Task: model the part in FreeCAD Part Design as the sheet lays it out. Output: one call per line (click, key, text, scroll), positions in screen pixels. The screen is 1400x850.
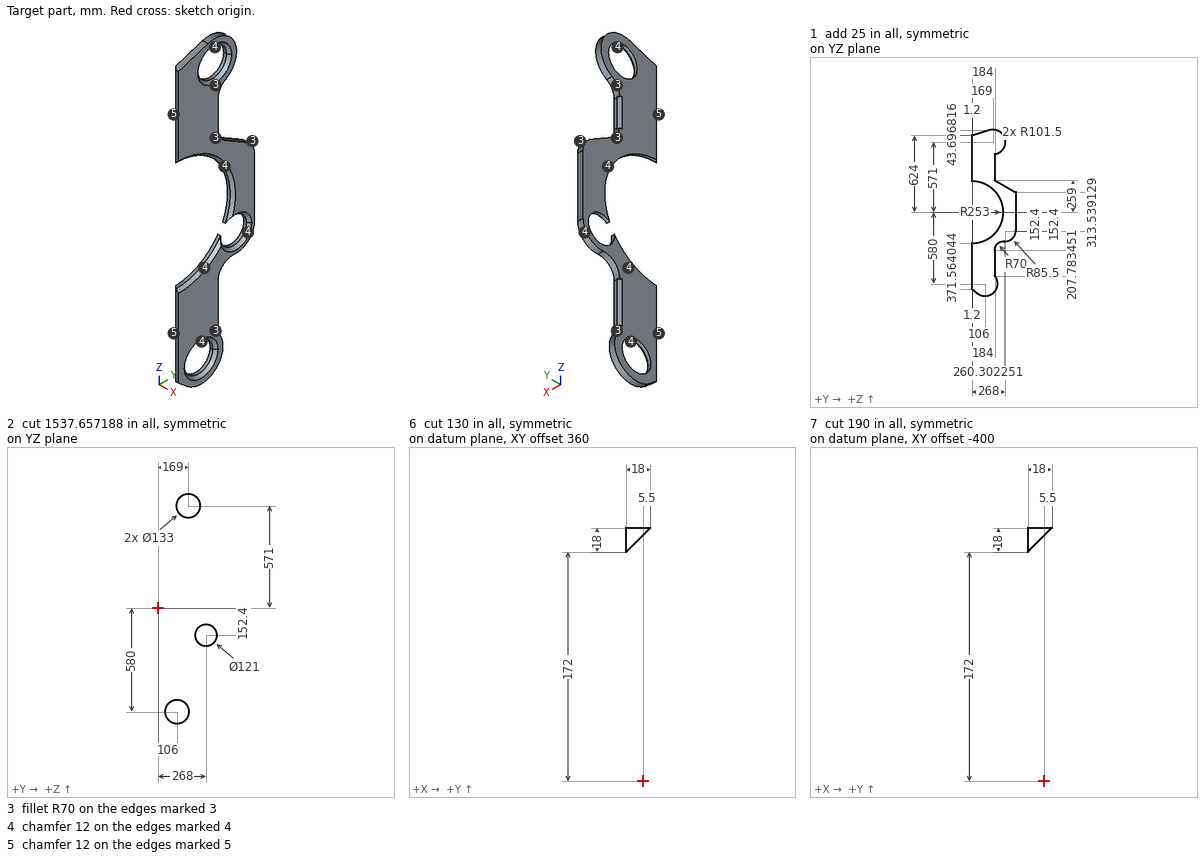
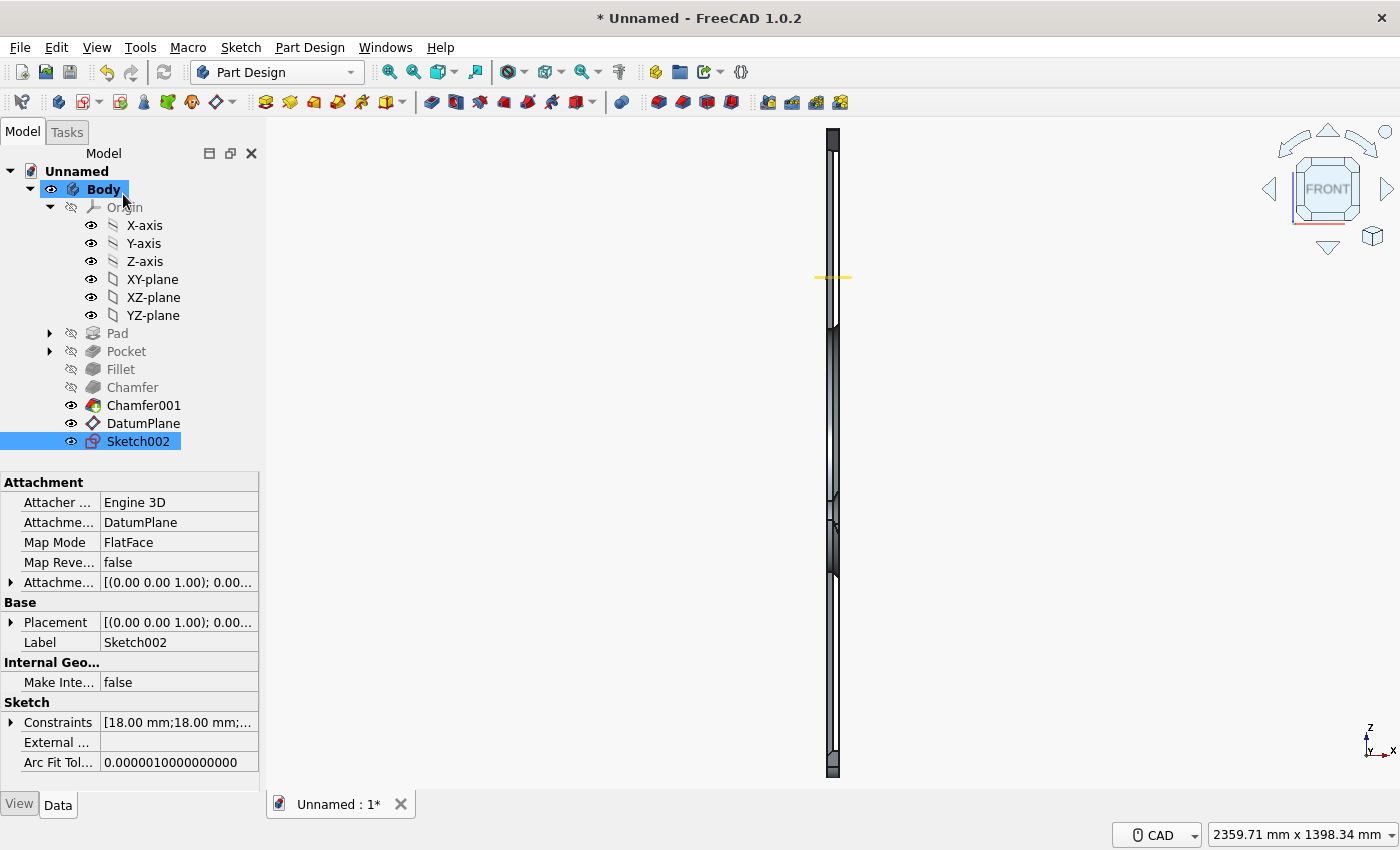
click(432, 102)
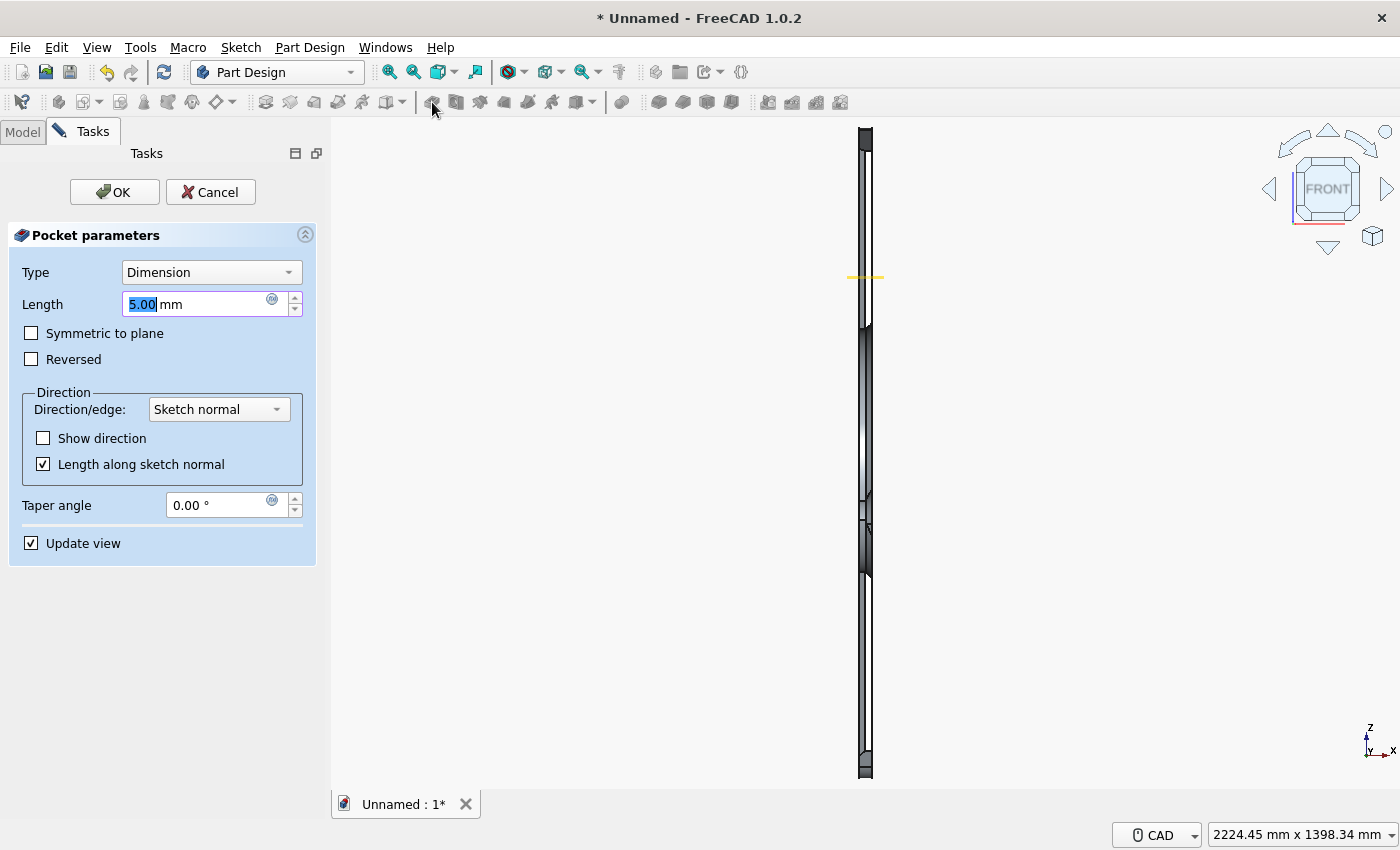
text(130)
key(Tab)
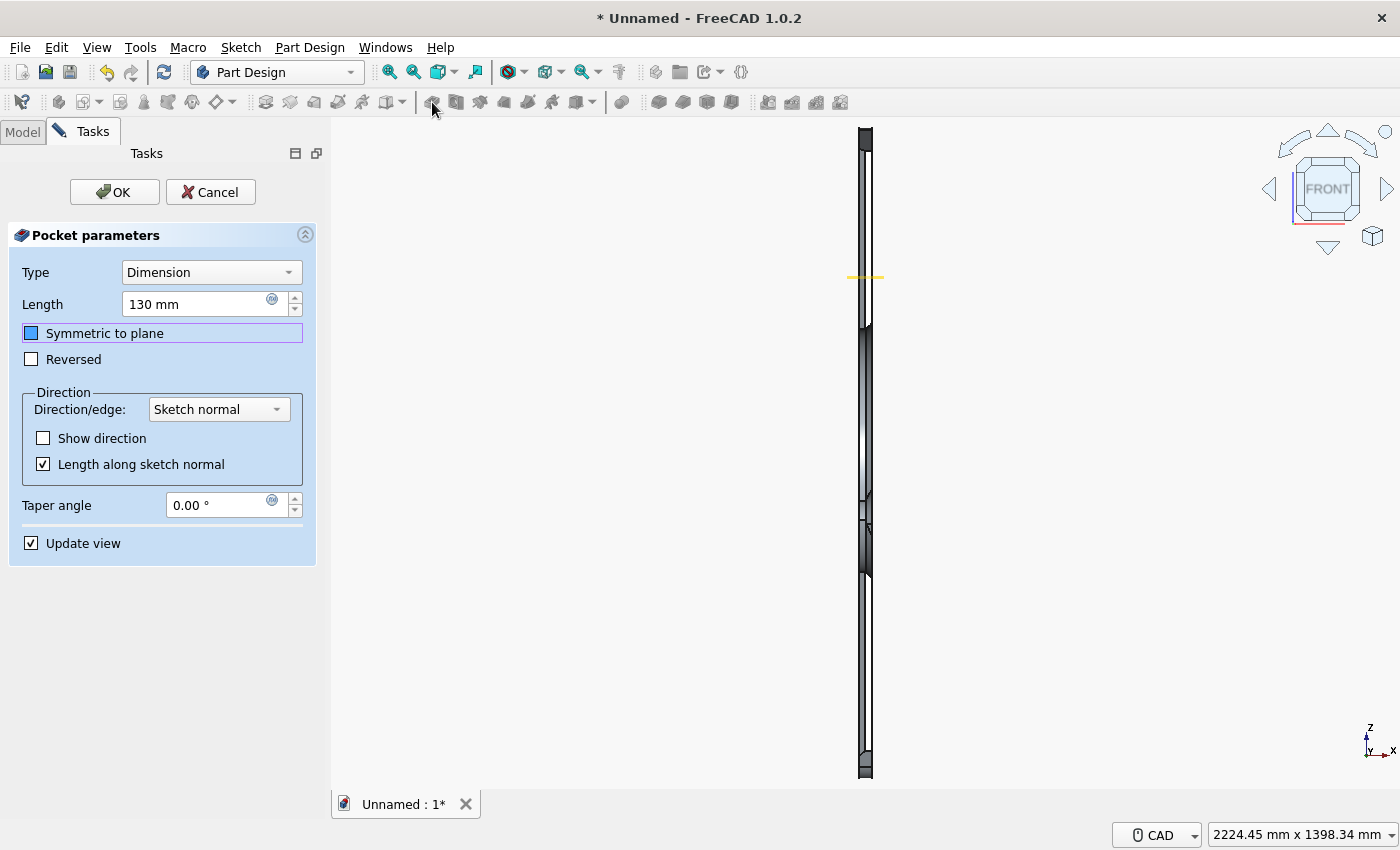
click(30, 333)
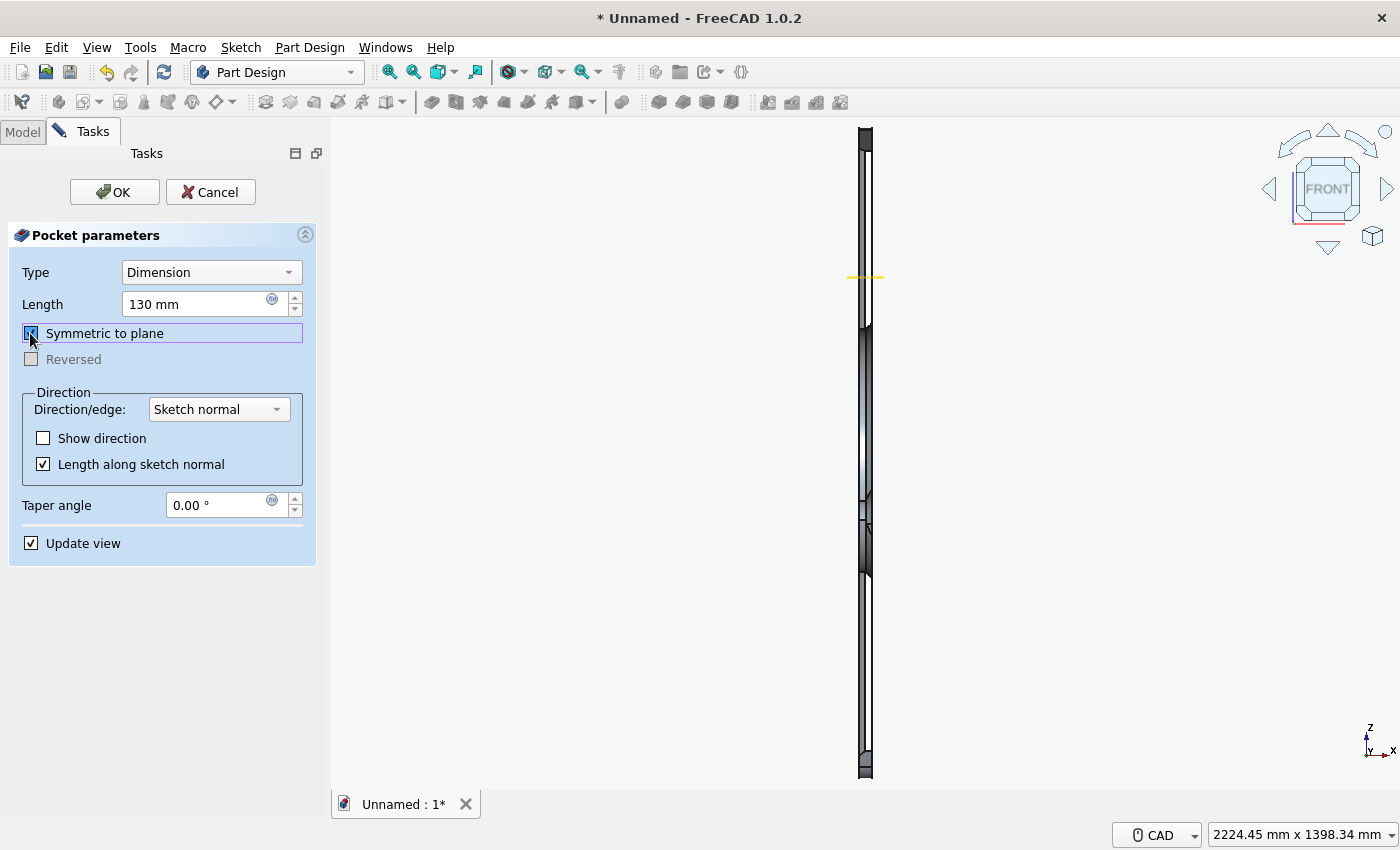
click(115, 192)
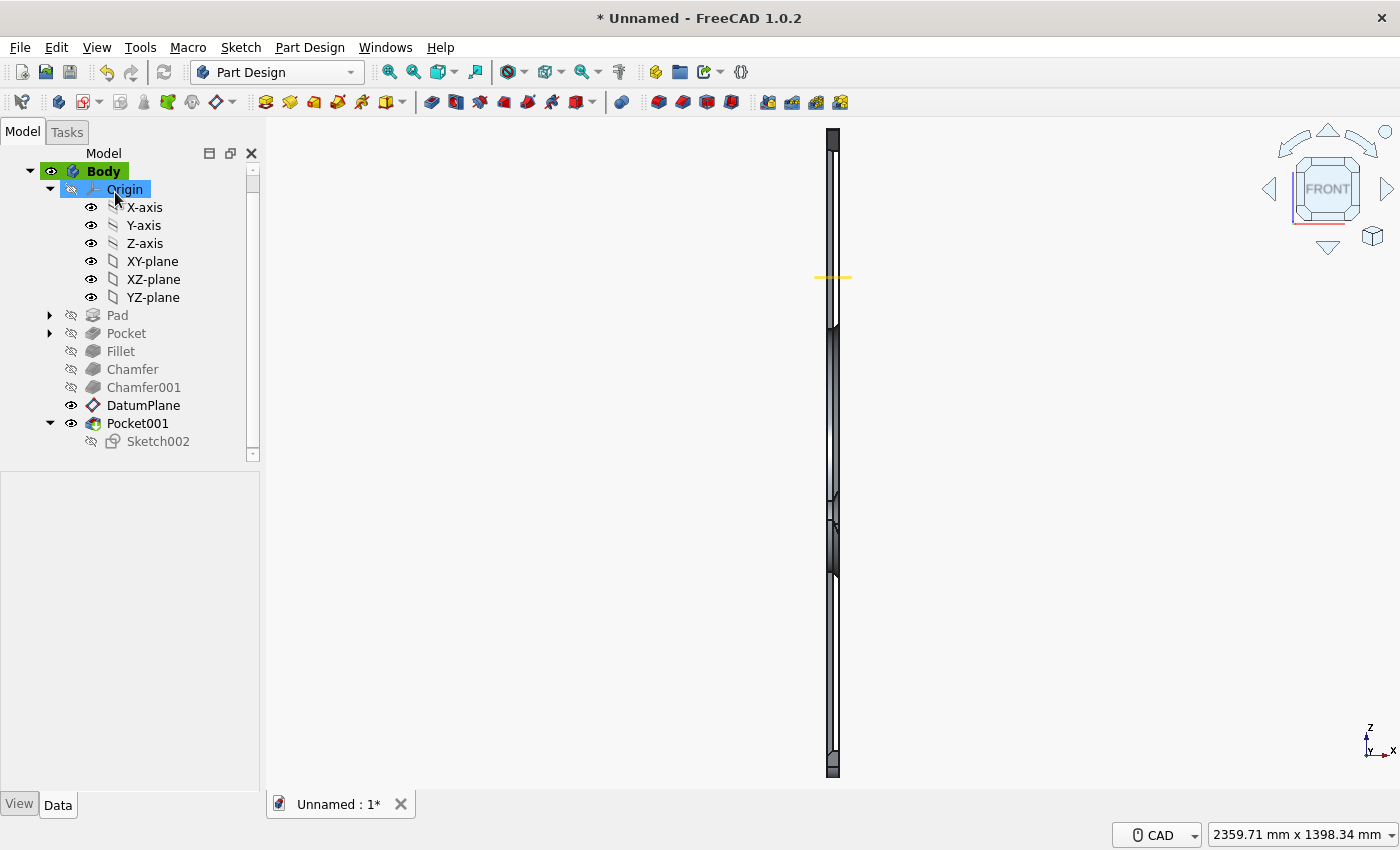
click(116, 405)
key(space)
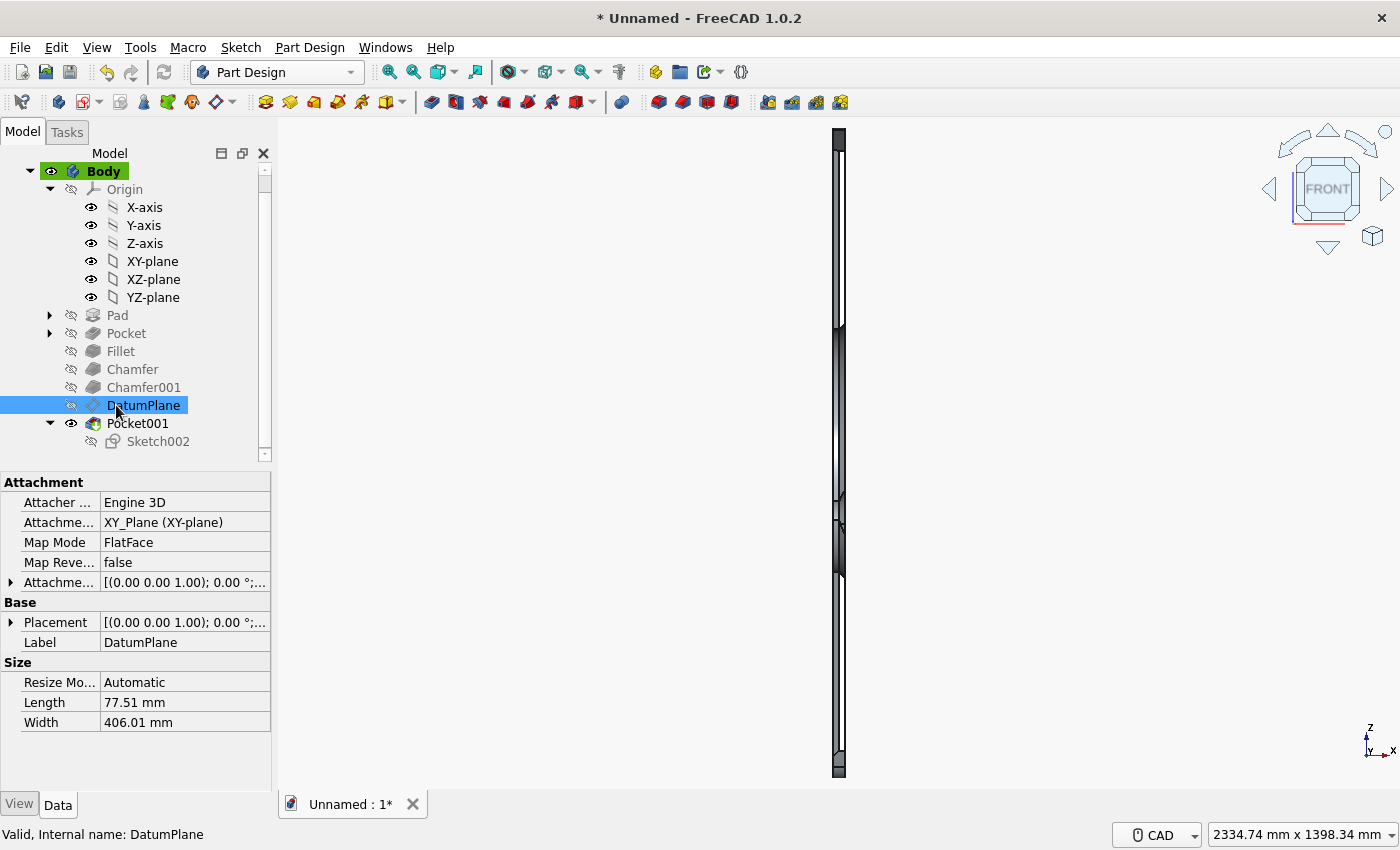
click(136, 261)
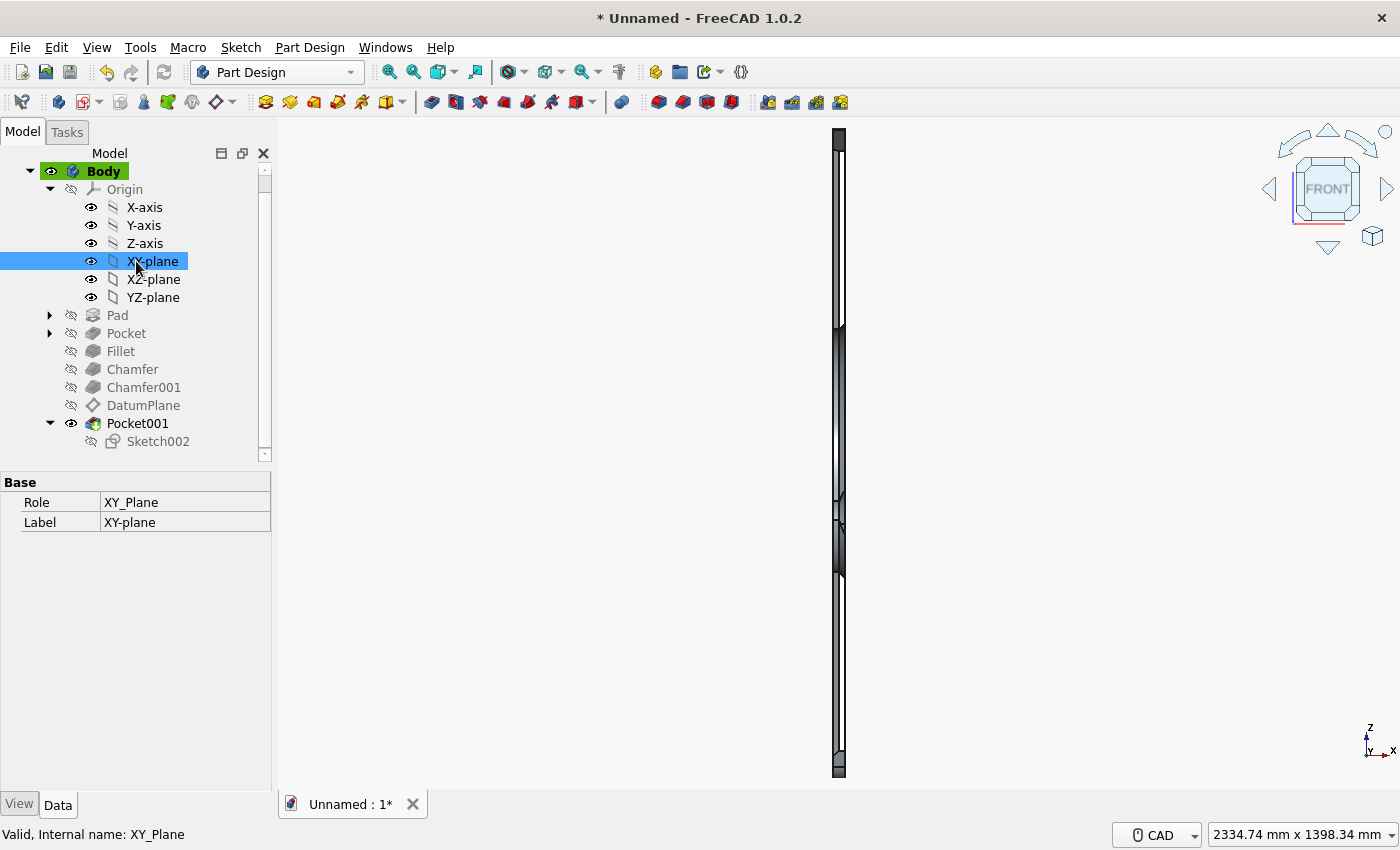
click(216, 102)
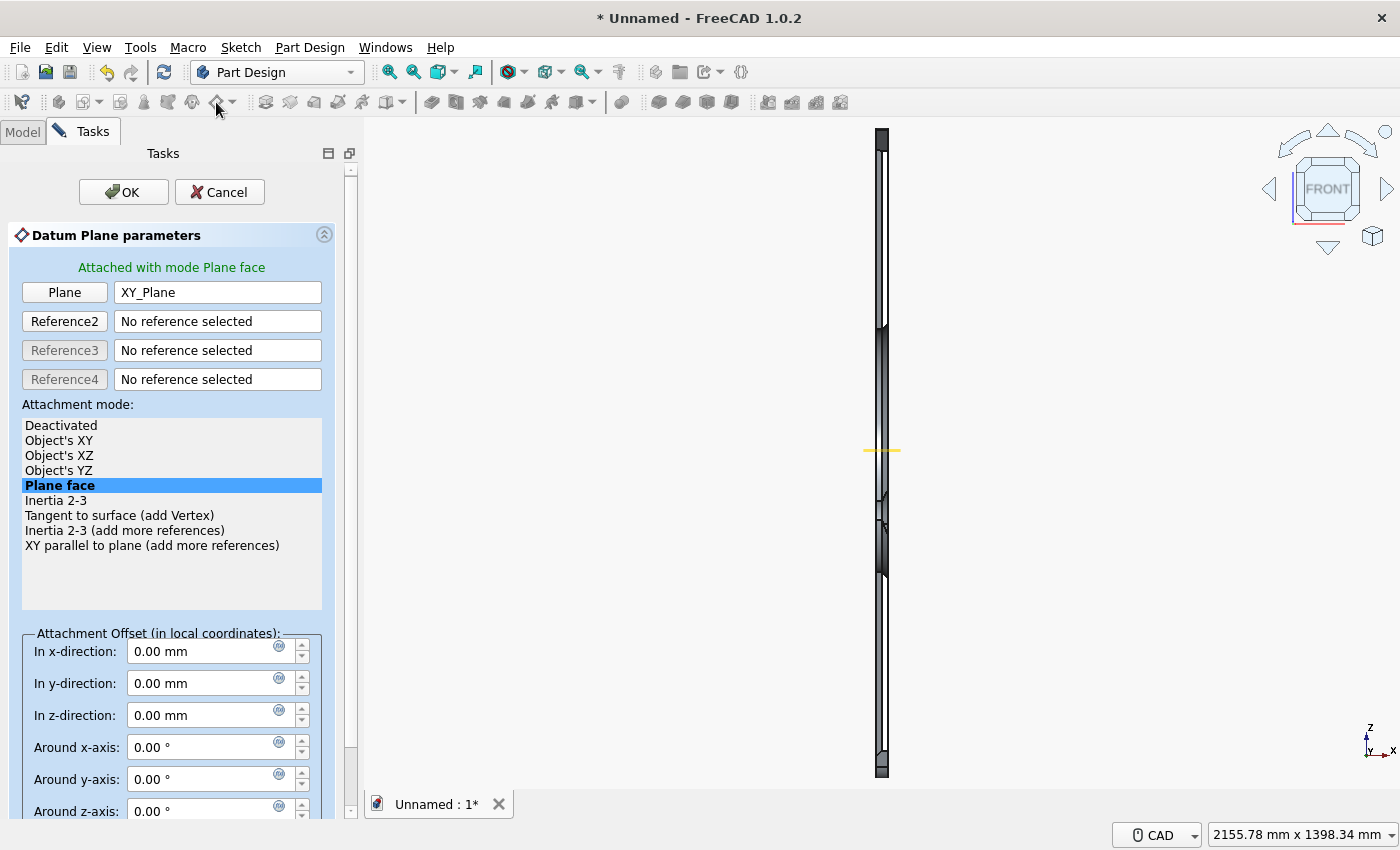
triple_click(210, 715)